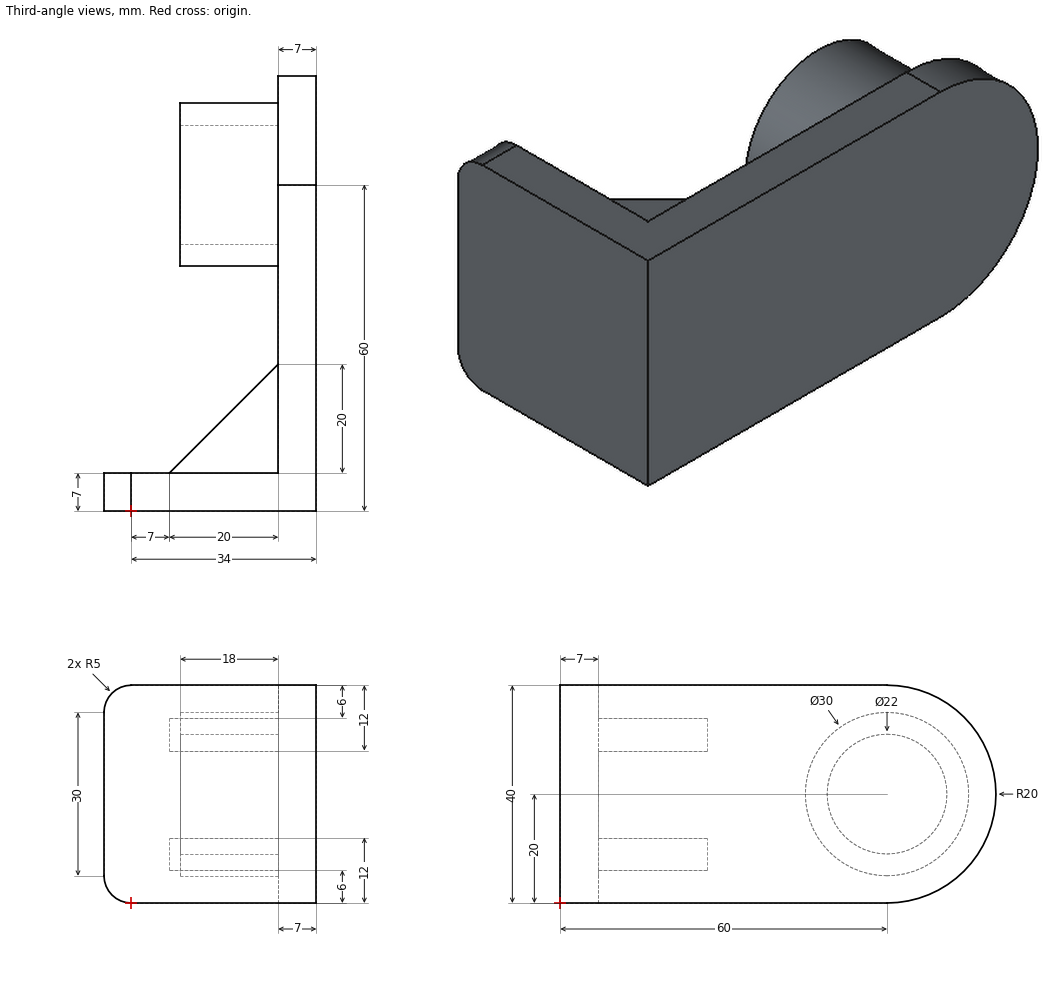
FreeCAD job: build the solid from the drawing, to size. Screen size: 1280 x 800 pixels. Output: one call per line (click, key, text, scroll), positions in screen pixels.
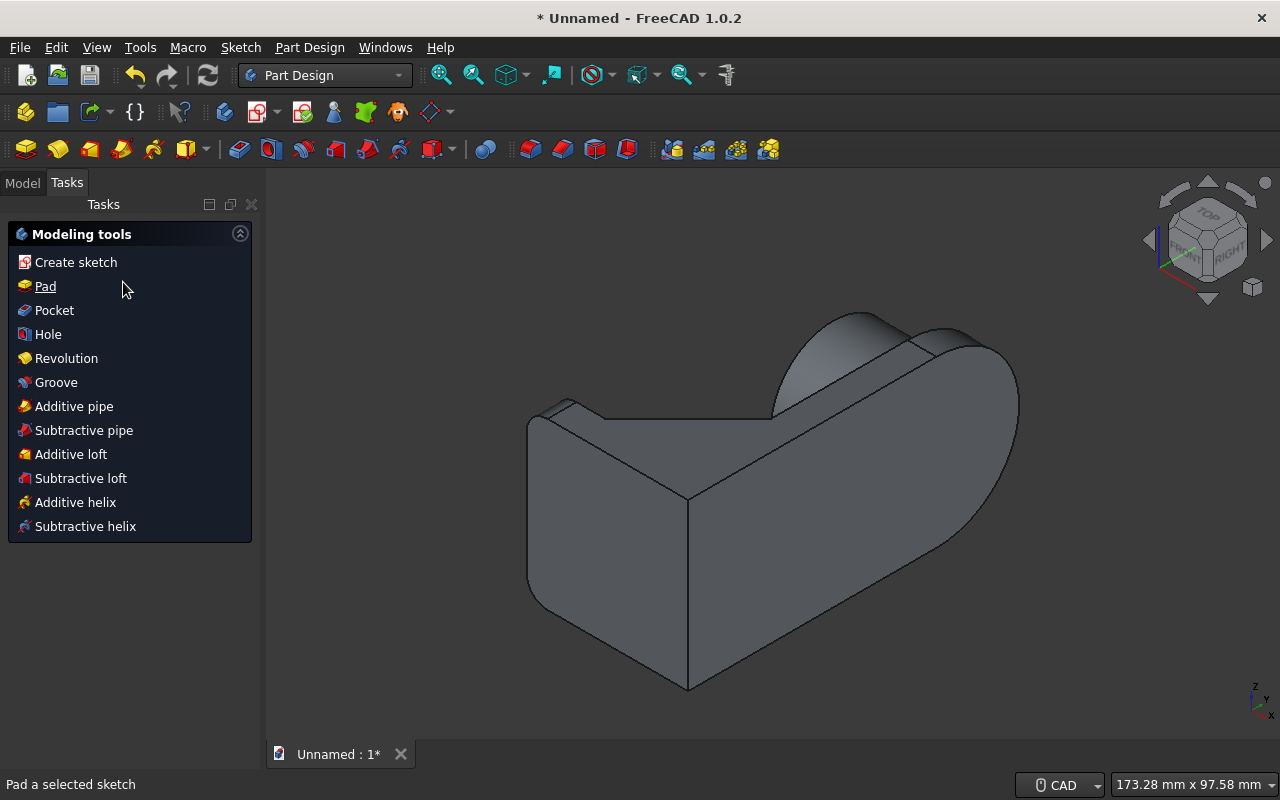
click(26, 150)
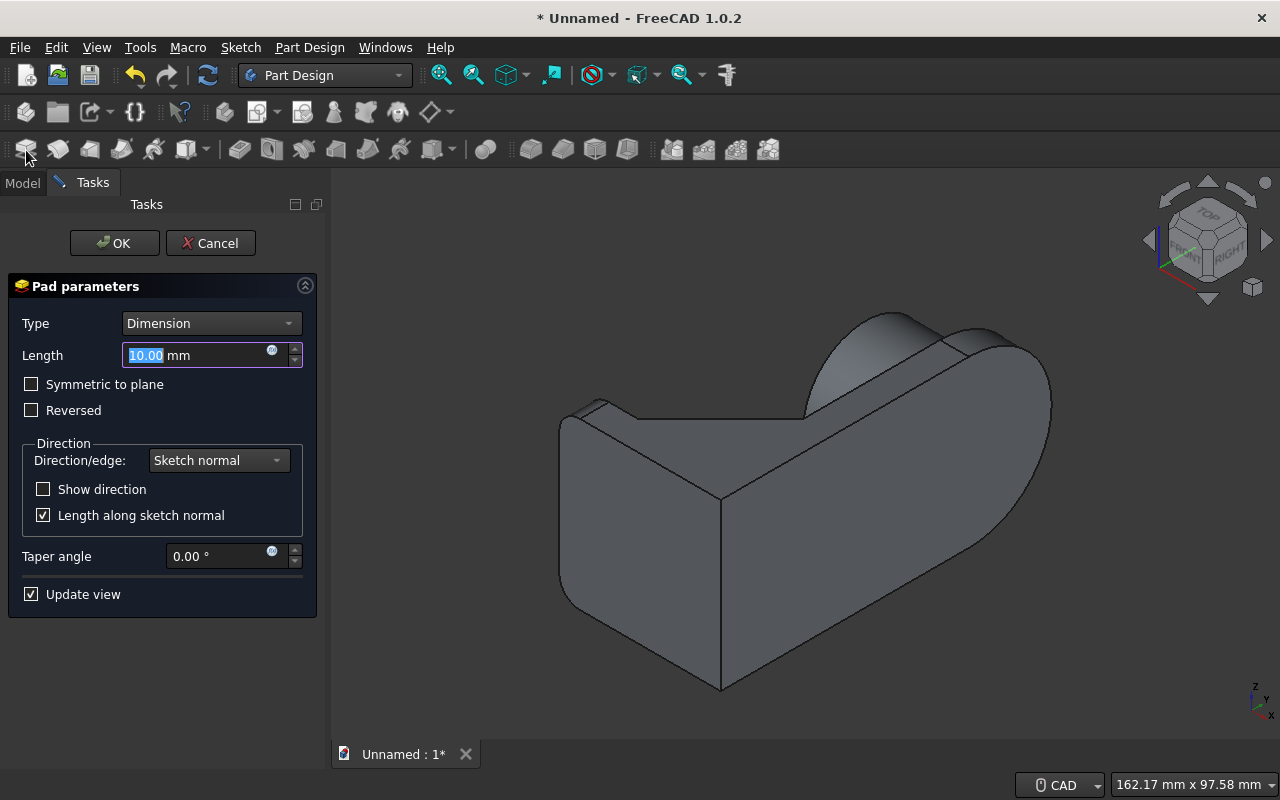
text(12)
key(Tab)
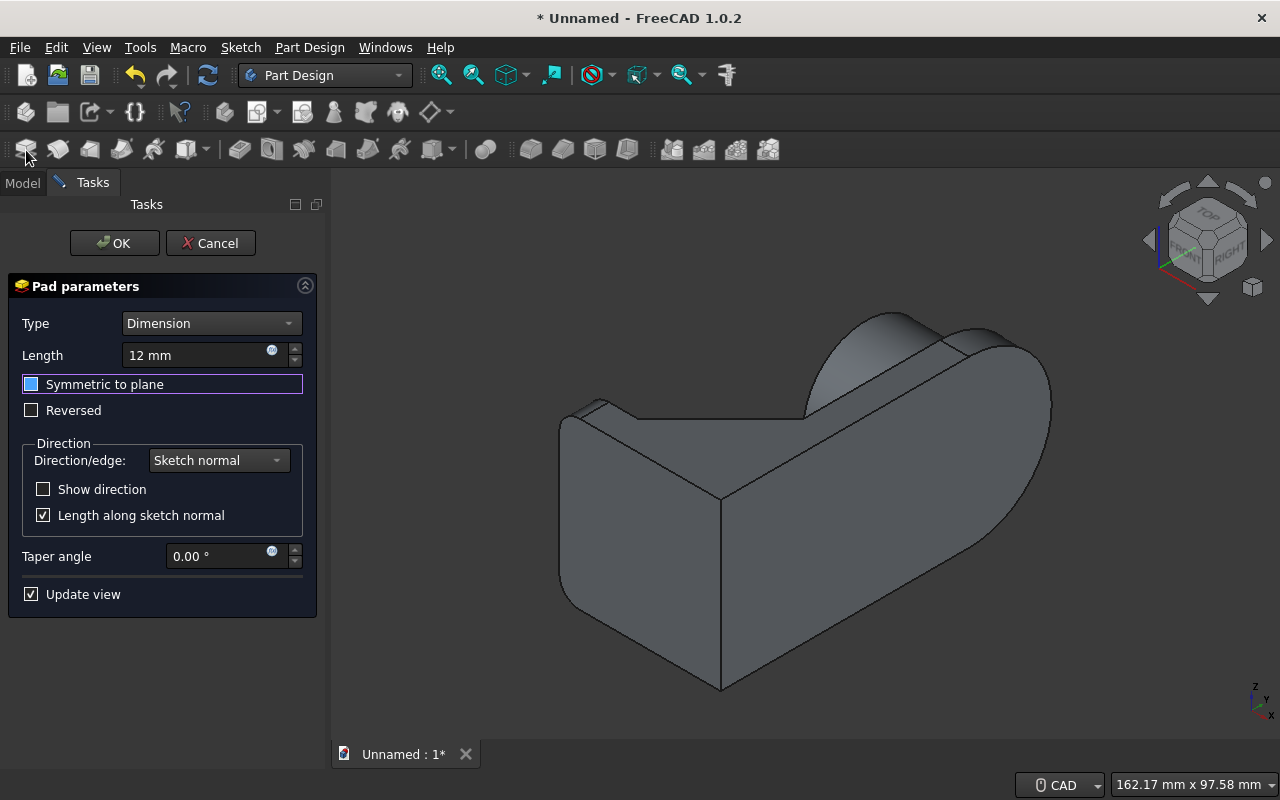
click(115, 243)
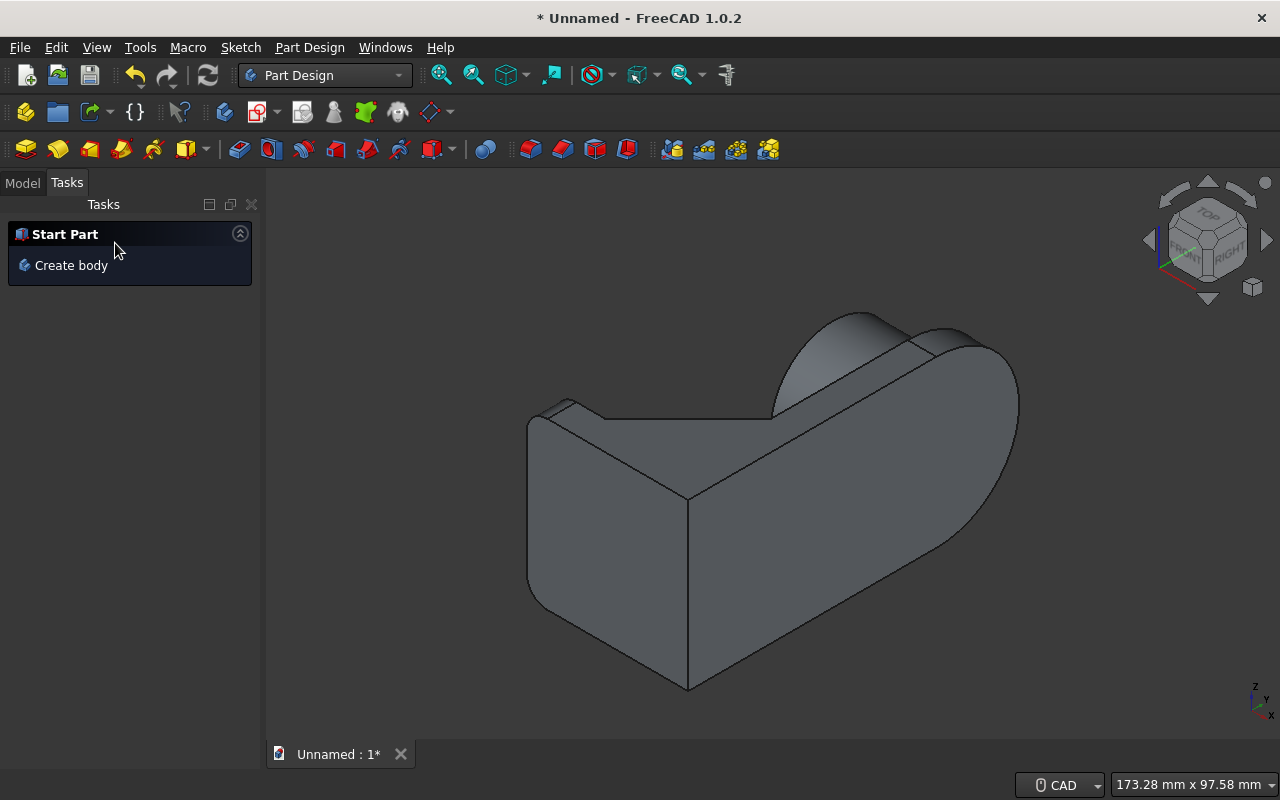
click(258, 112)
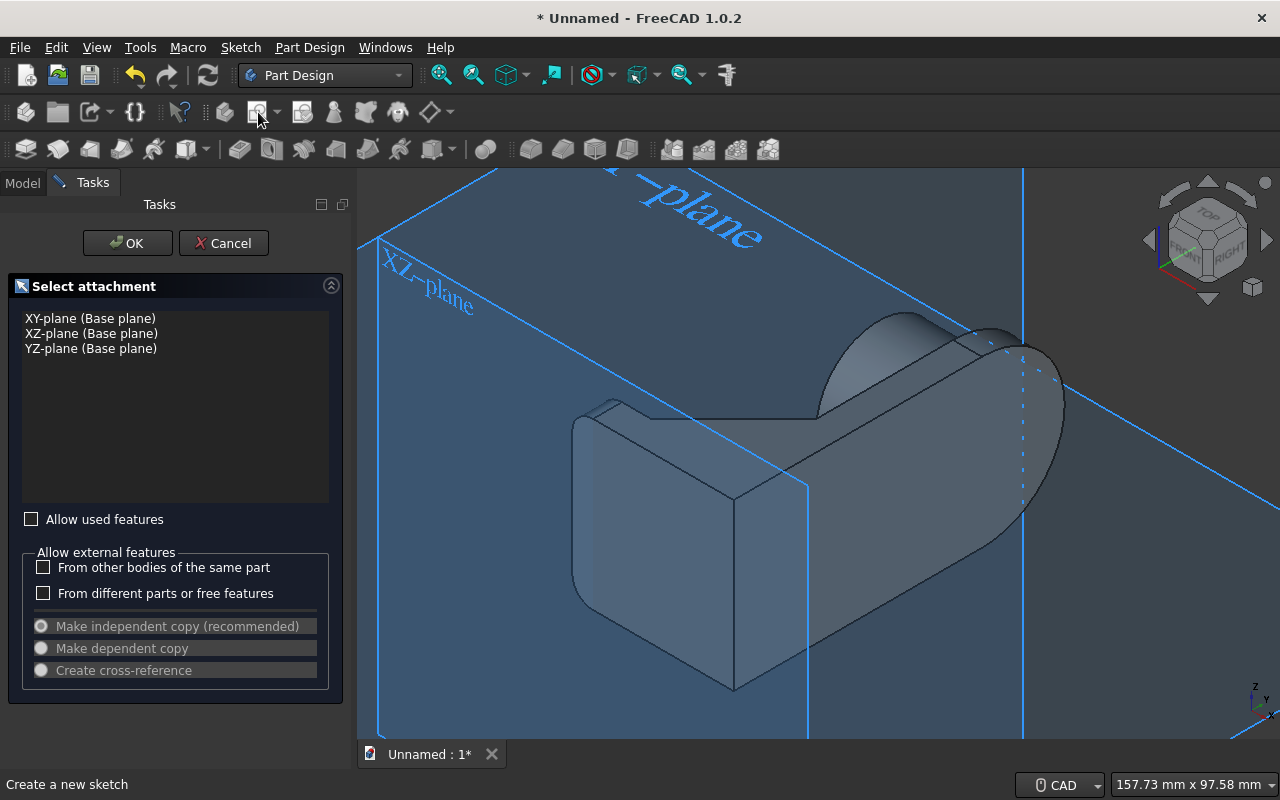
click(82, 318)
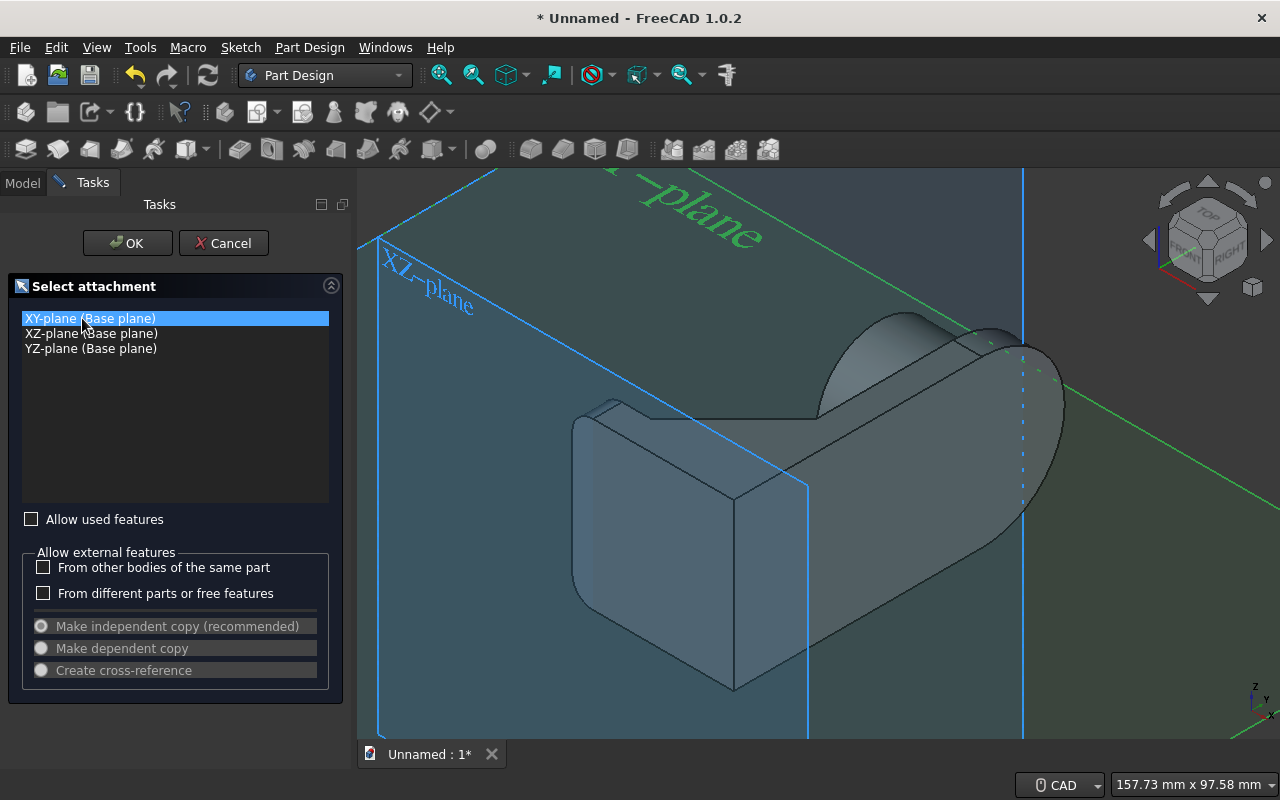
click(128, 243)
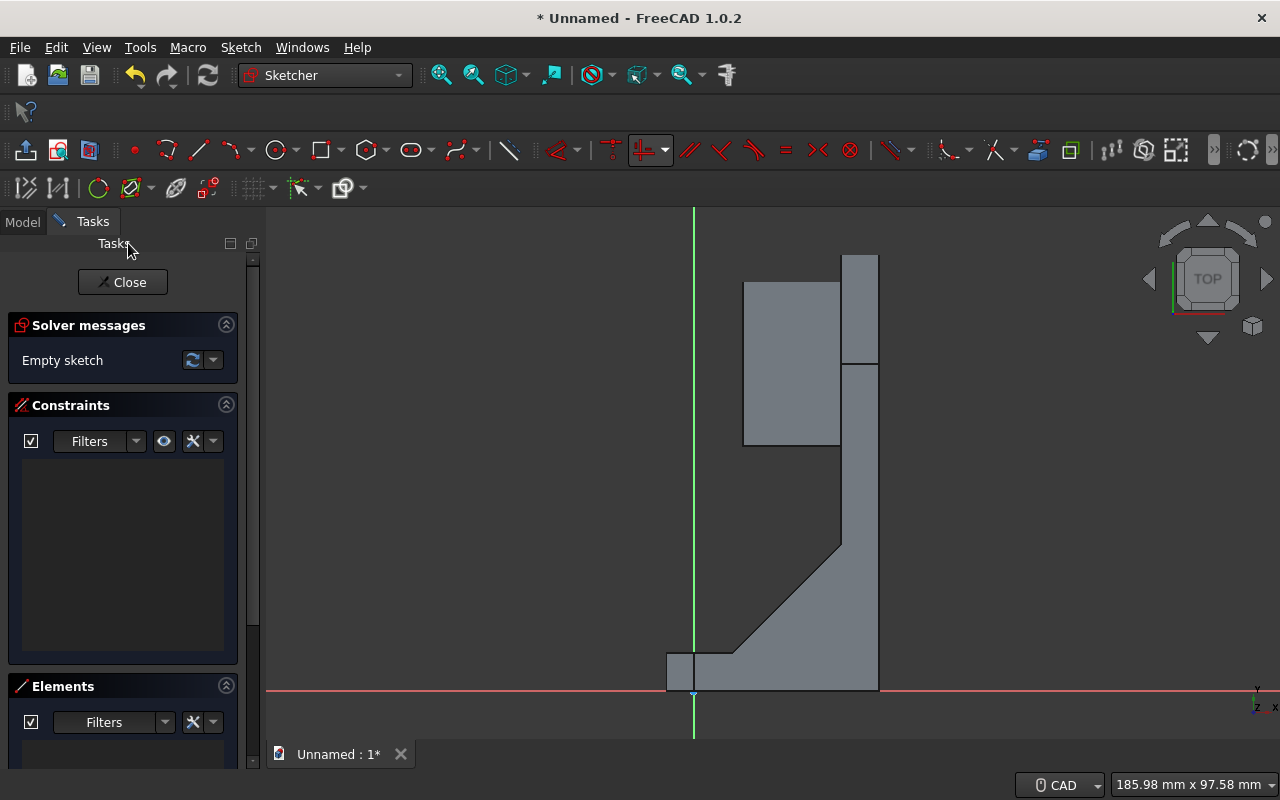
click(90, 150)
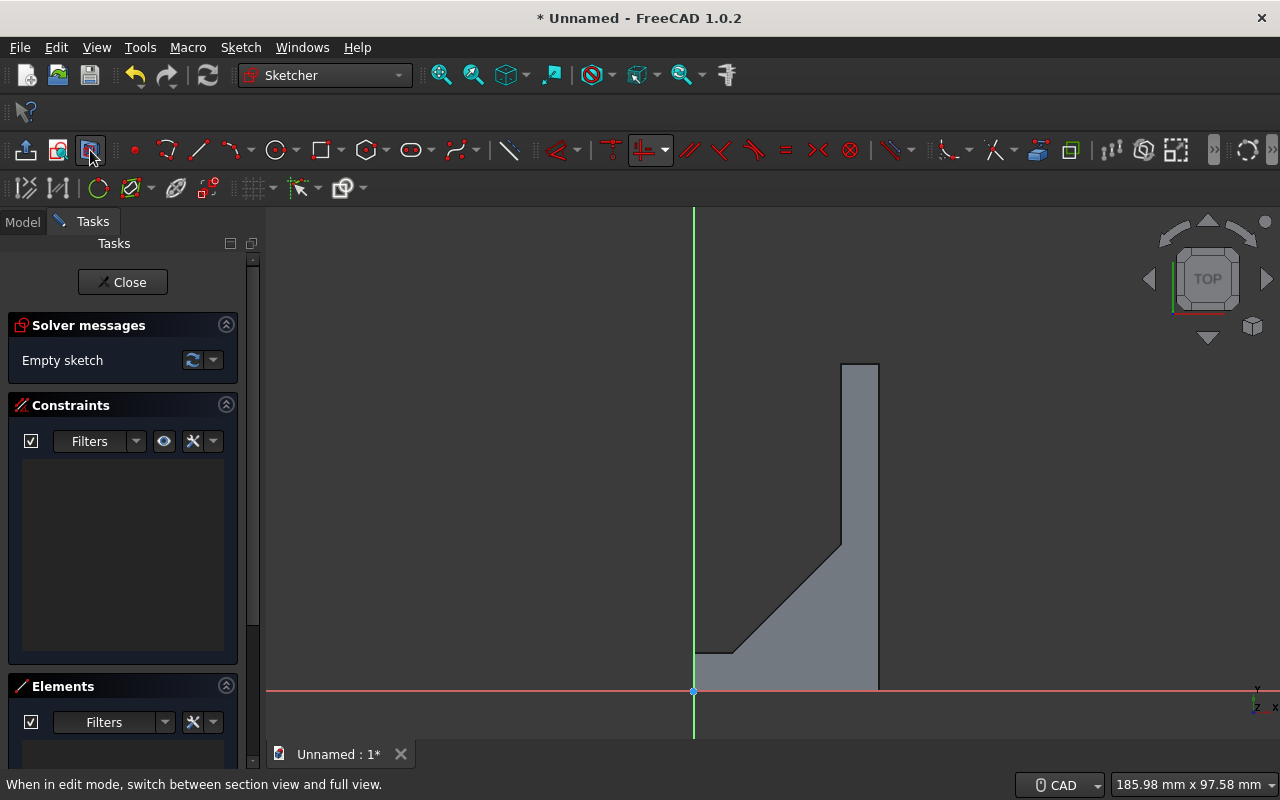
scroll(819, 711, up, 4)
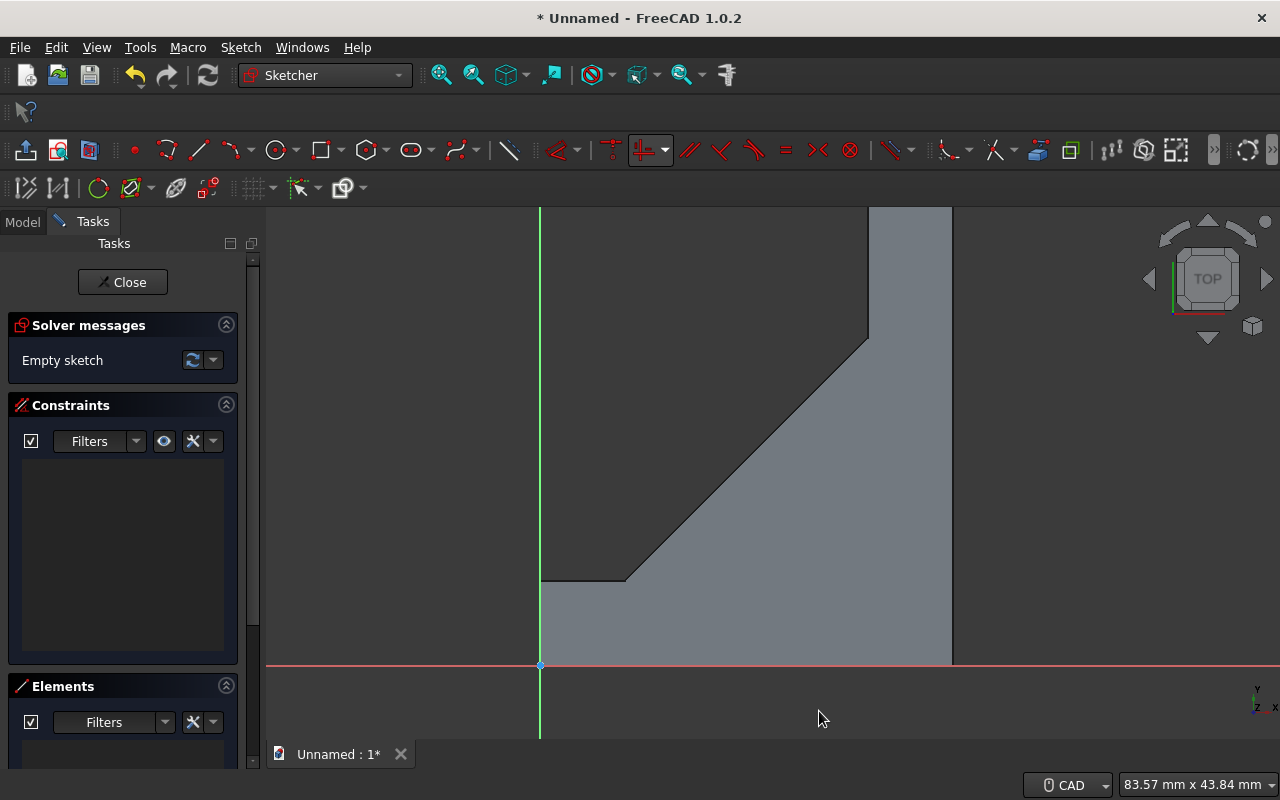
click(168, 150)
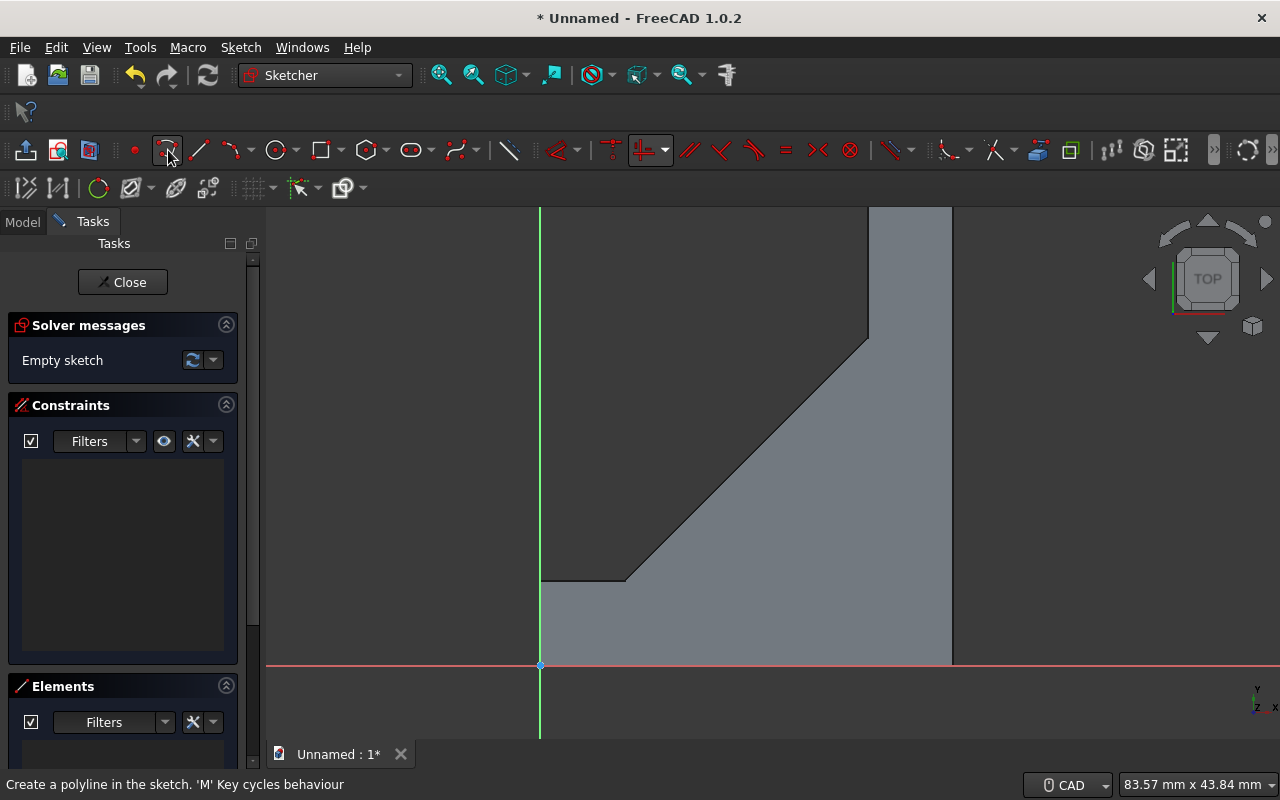
click(625, 581)
click(868, 338)
click(868, 581)
click(625, 582)
key(Escape)
key(Escape)